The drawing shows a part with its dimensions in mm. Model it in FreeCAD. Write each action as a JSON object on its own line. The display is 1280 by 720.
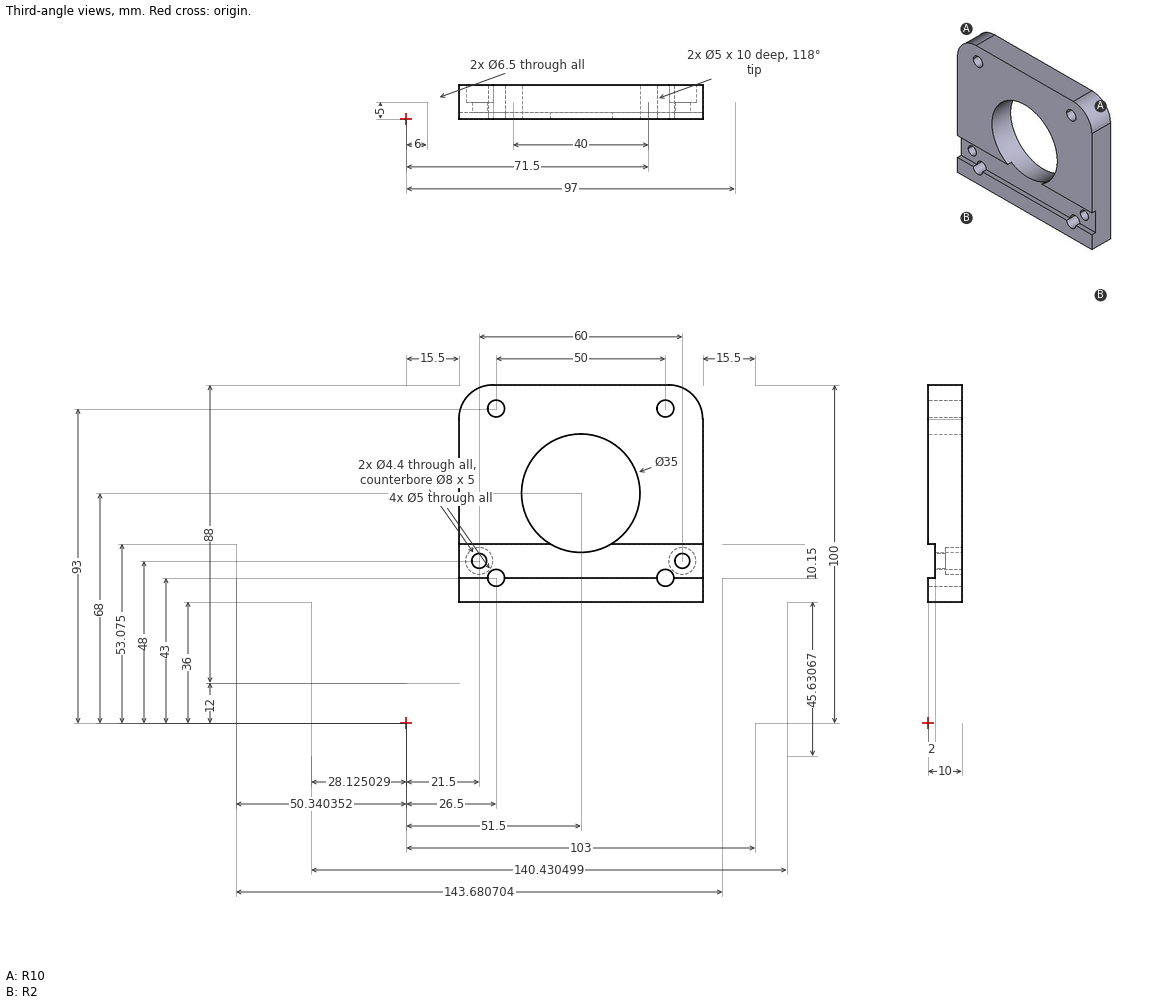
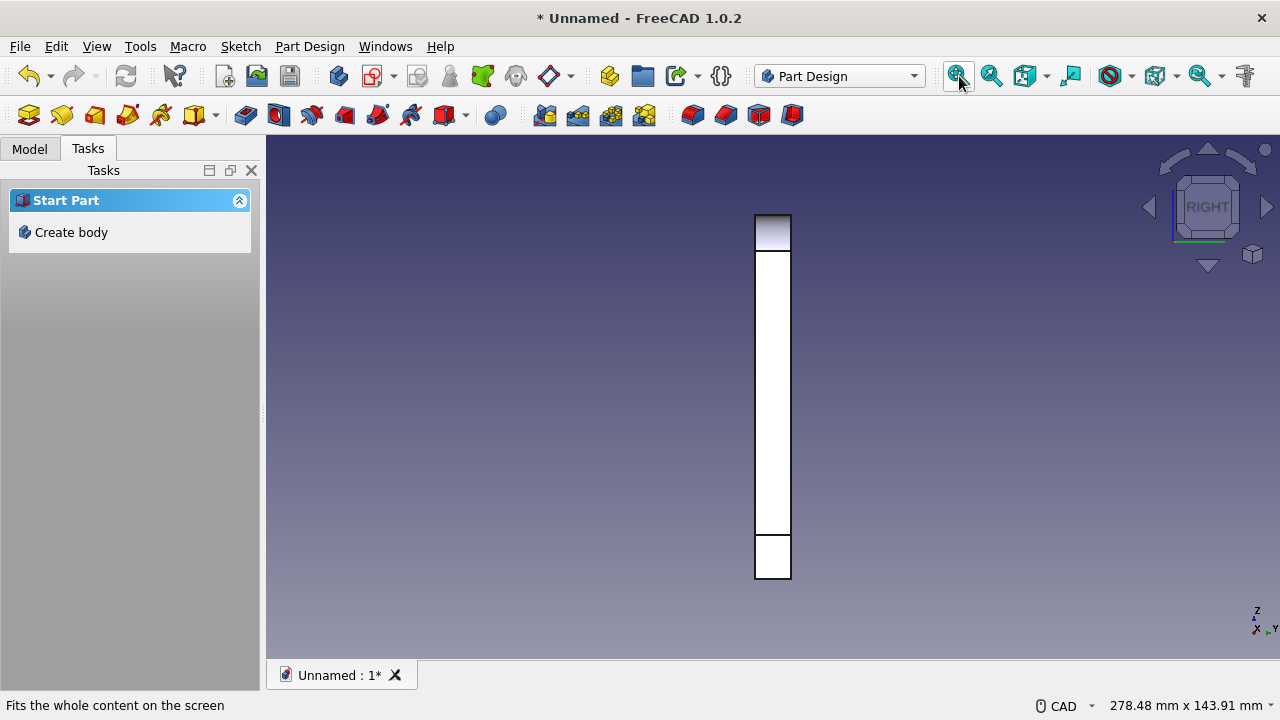
{"action": "key", "text": "5"}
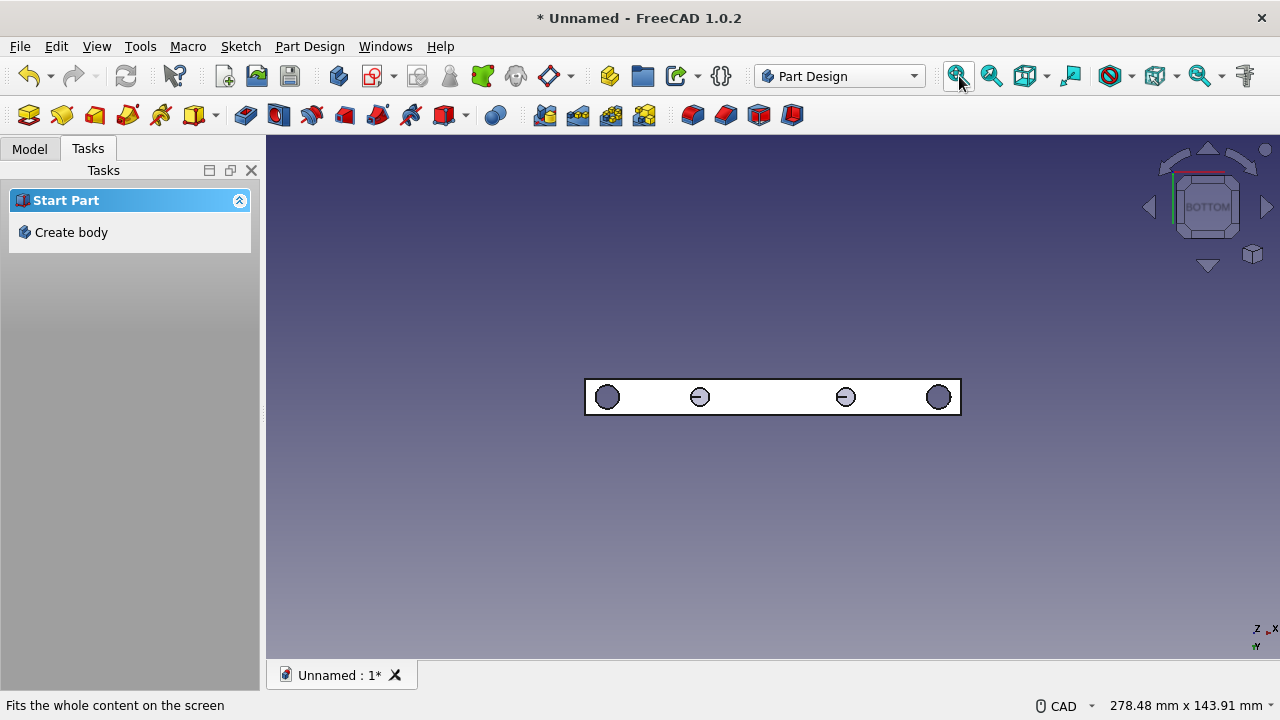
{"action": "left_click", "coordinate": [959, 76]}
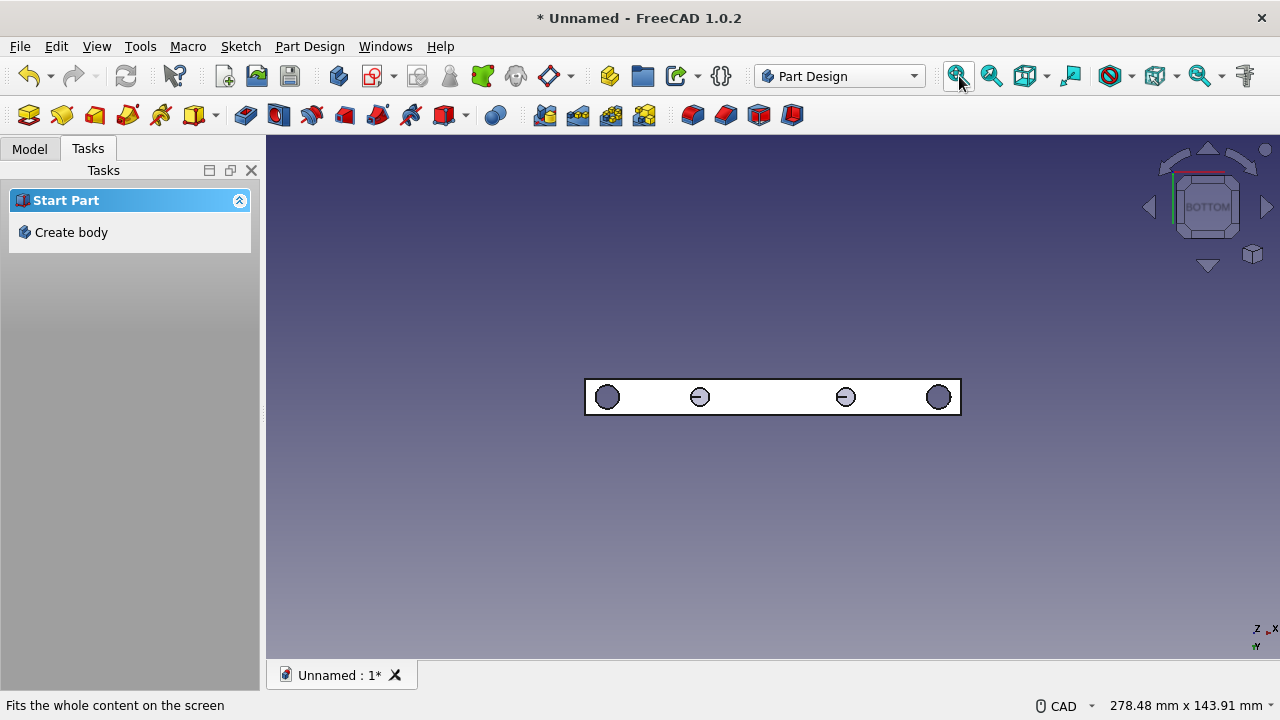
{"action": "key", "text": "4"}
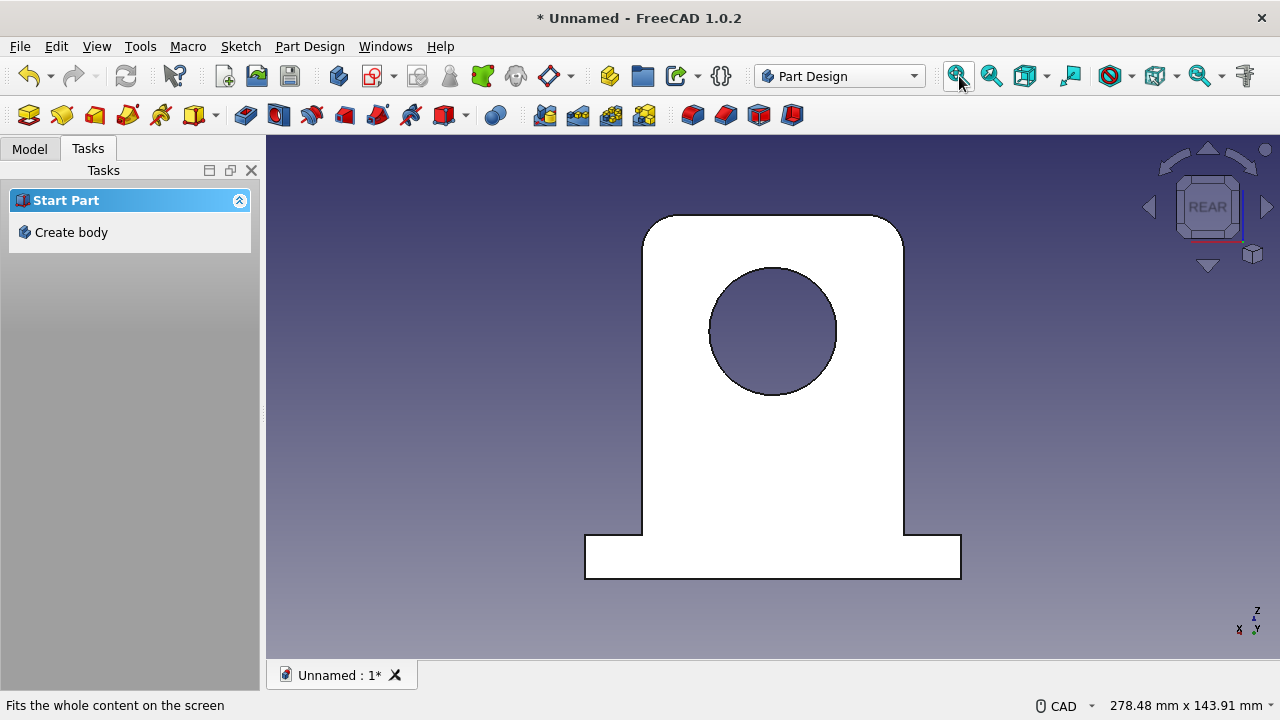
{"action": "key", "text": "6"}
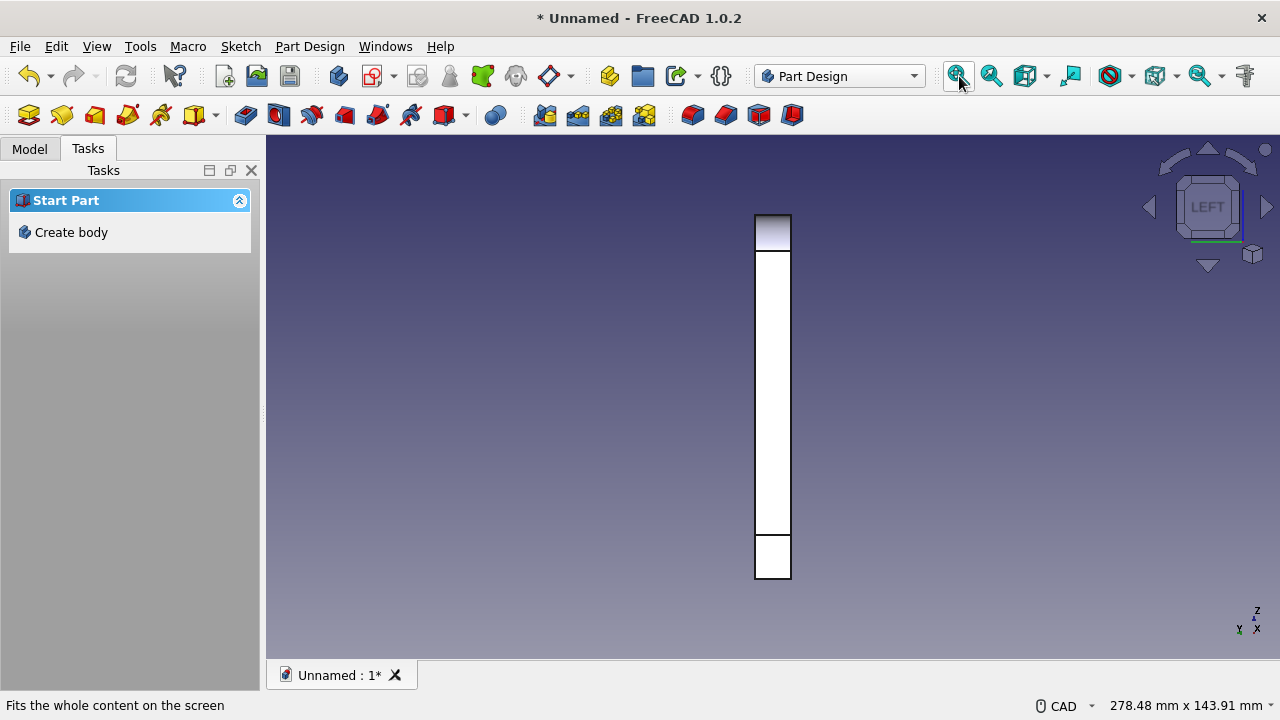
{"action": "key", "text": "v 3"}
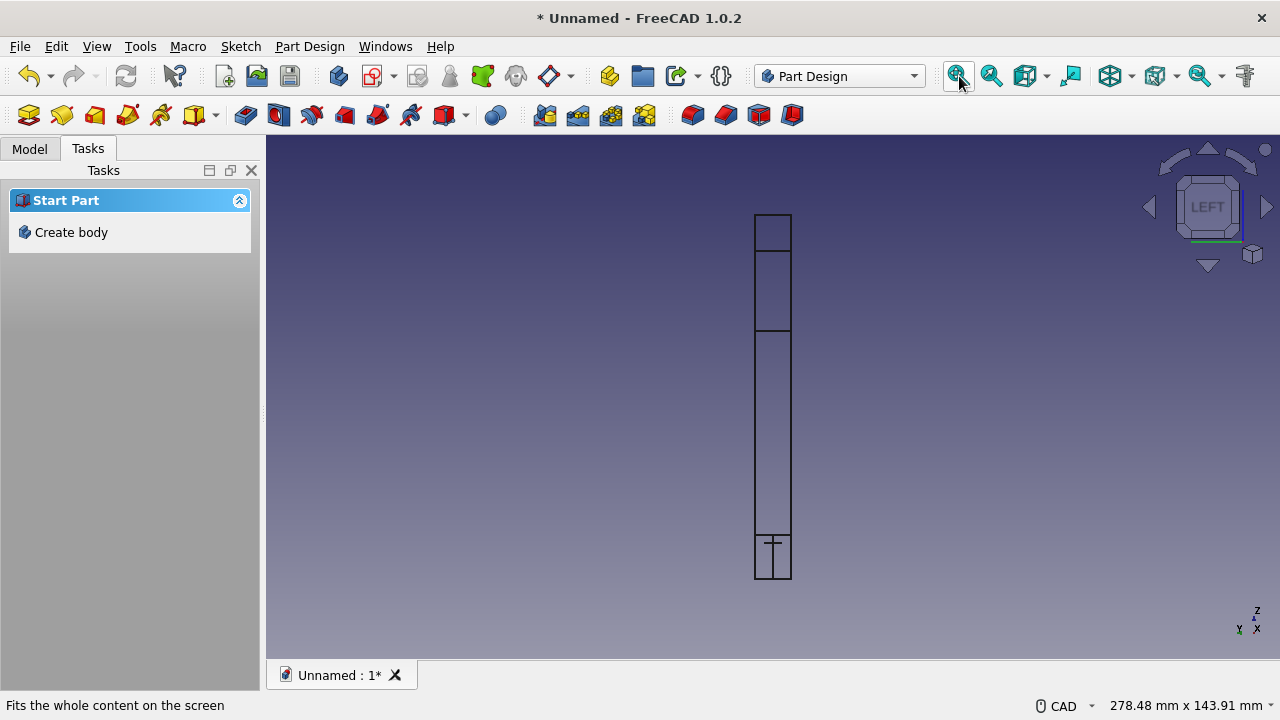
{"action": "key", "text": "0"}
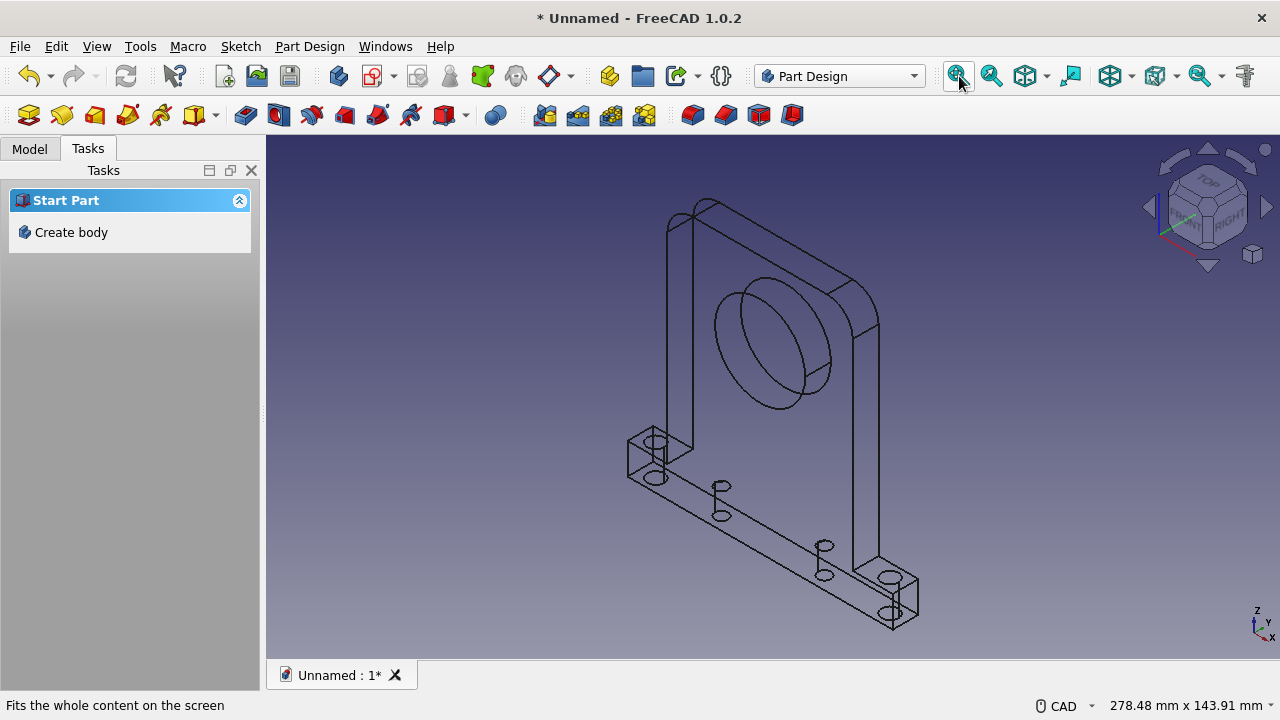
{"action": "left_click", "coordinate": [680, 455]}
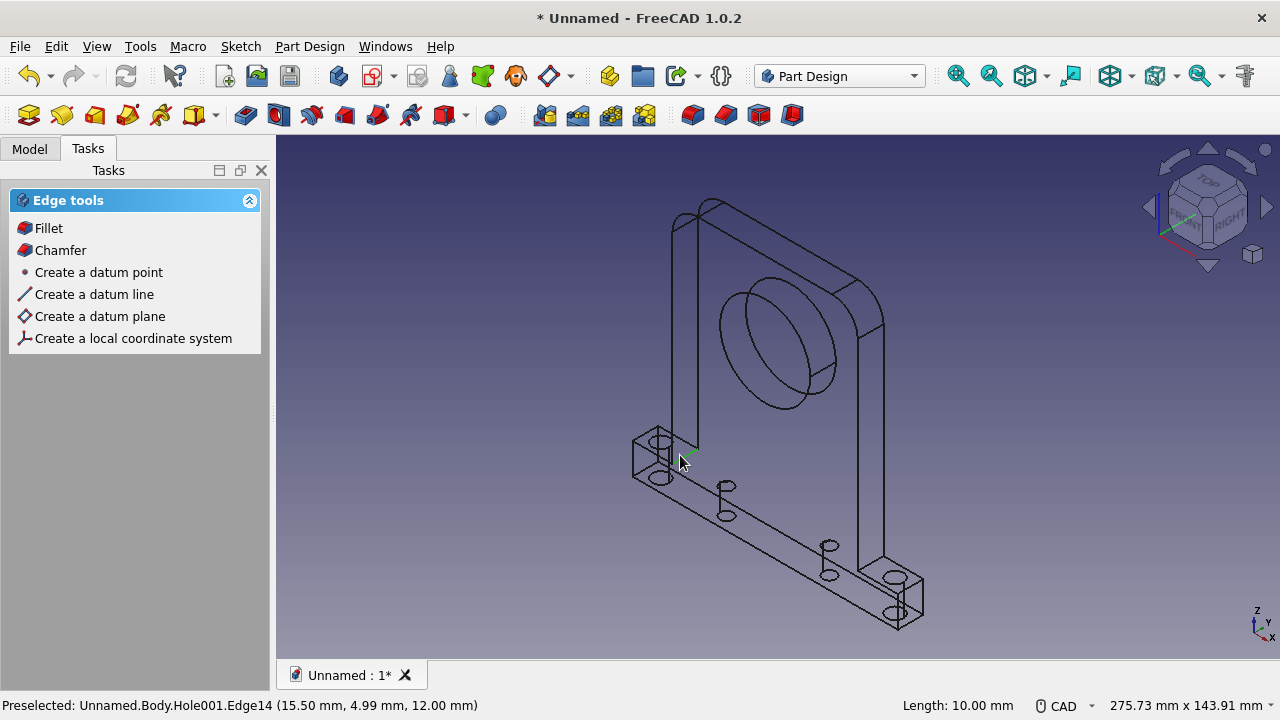
{"action": "left_click", "coordinate": [871, 562], "text": "ctrl"}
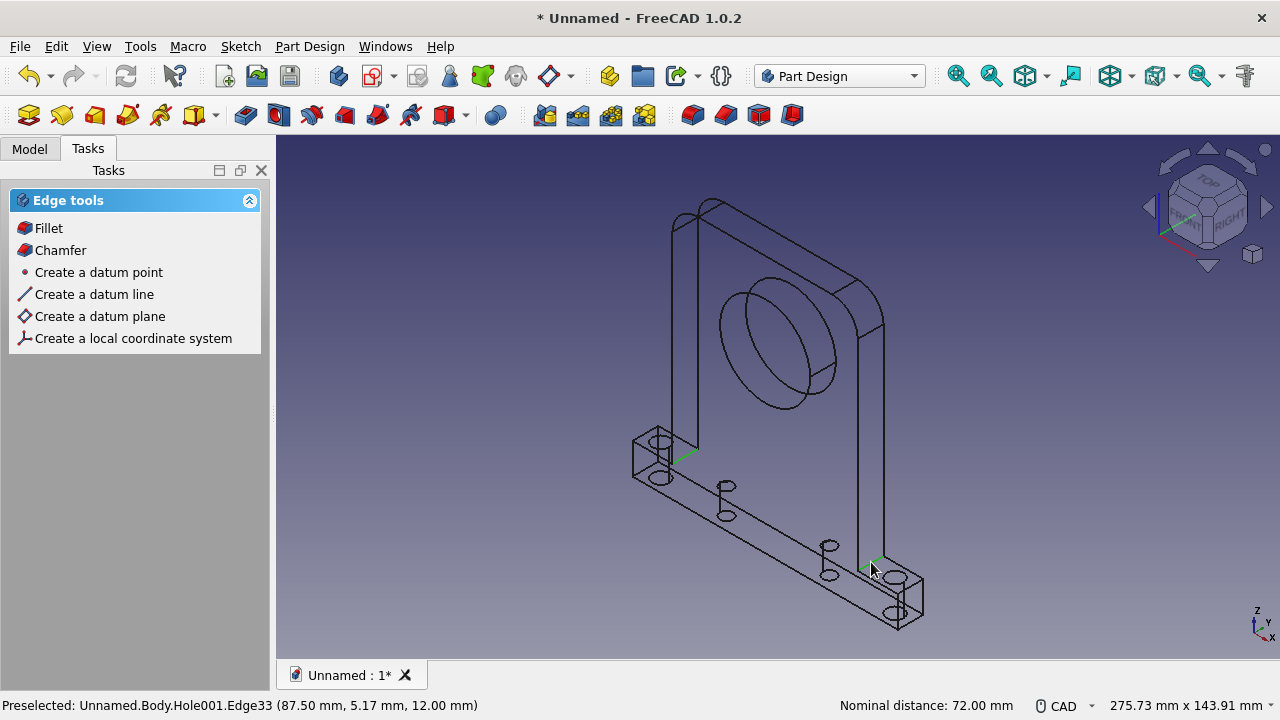
{"action": "key", "text": "v 1"}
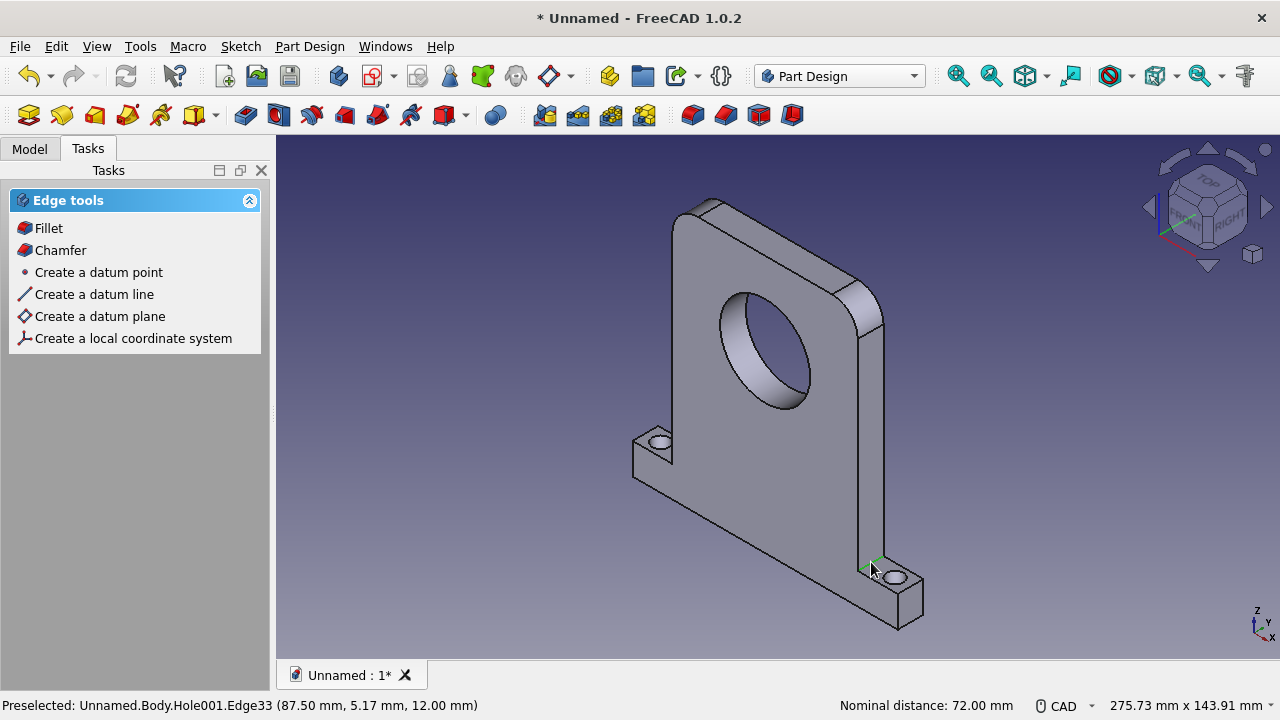
{"action": "left_click", "coordinate": [693, 116]}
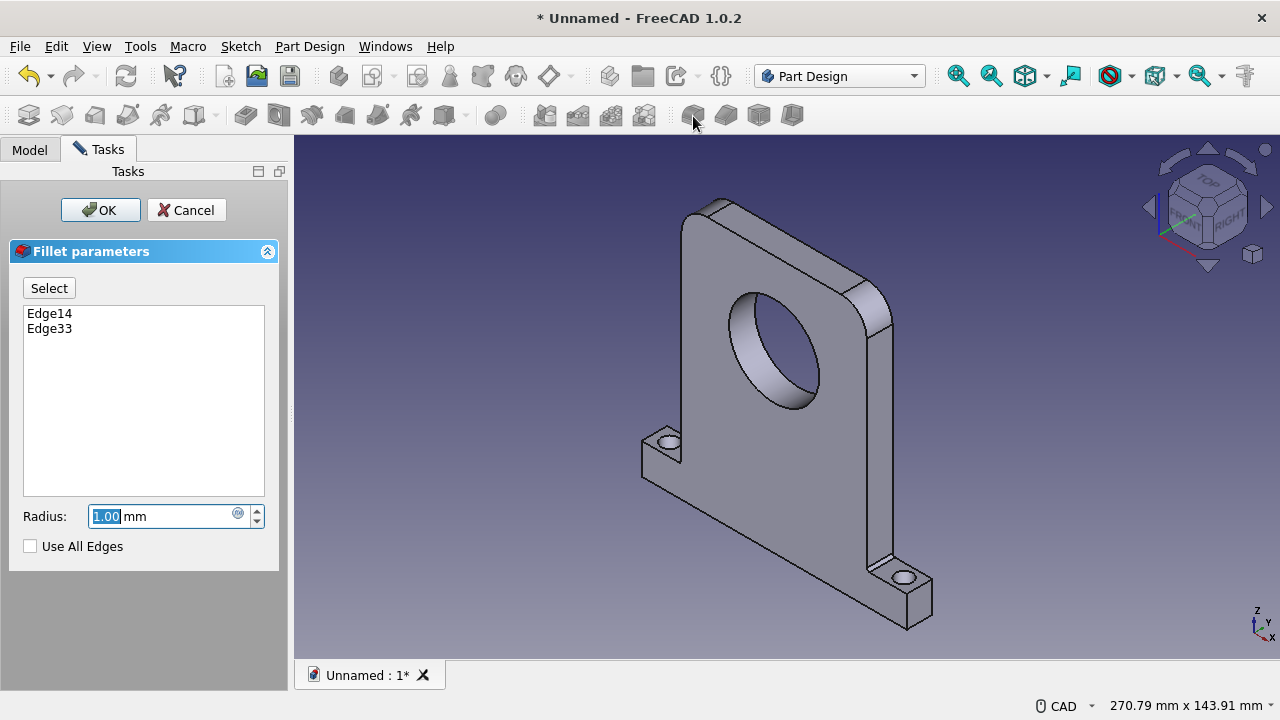
{"action": "type", "text": "2"}
{"action": "key", "text": "Tab"}